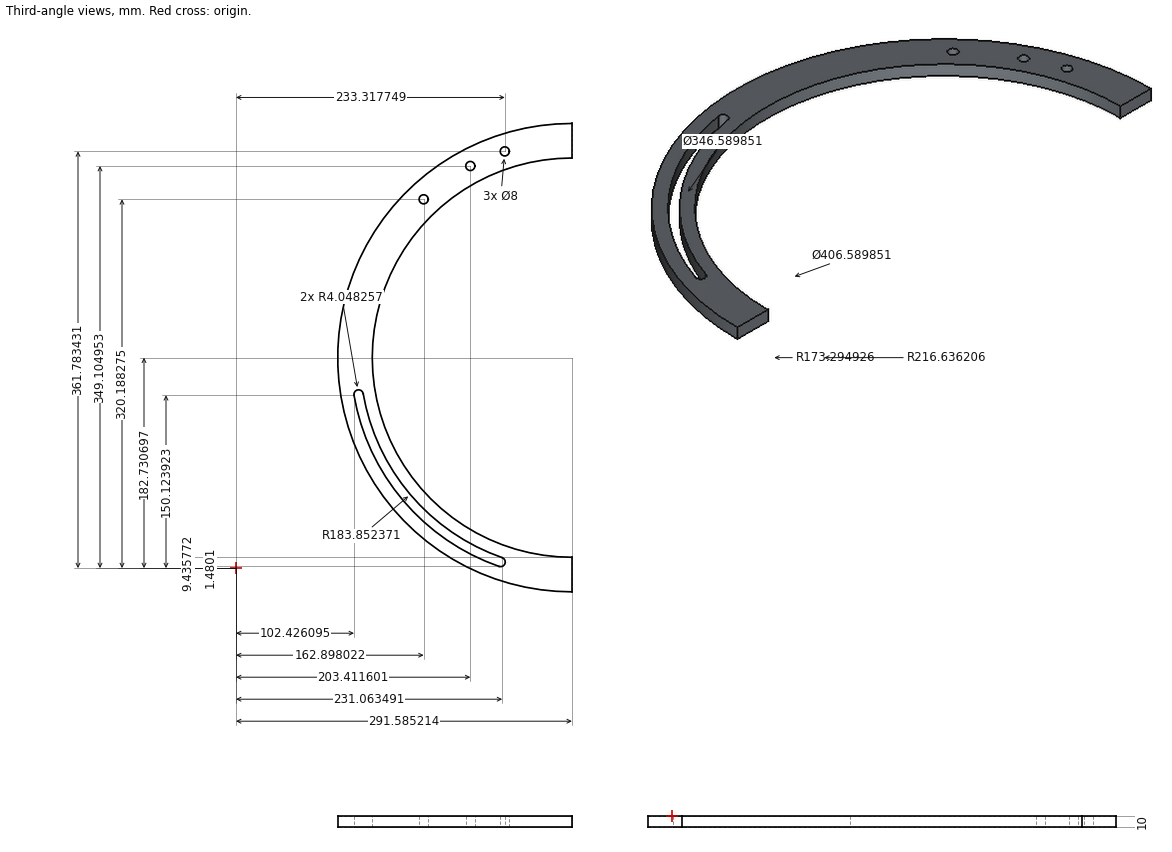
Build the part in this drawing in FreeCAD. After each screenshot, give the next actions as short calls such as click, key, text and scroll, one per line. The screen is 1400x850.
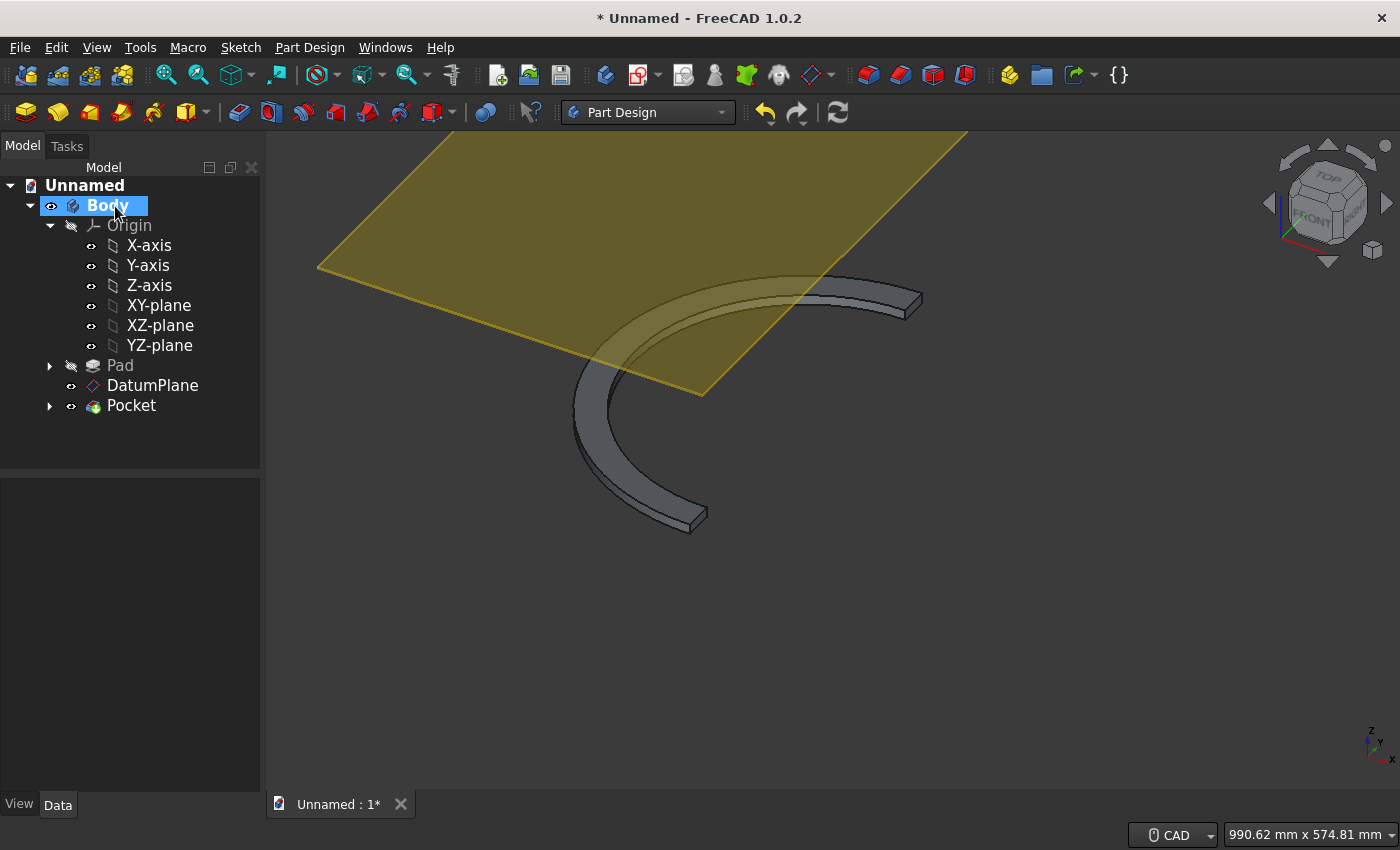
click(116, 386)
key(space)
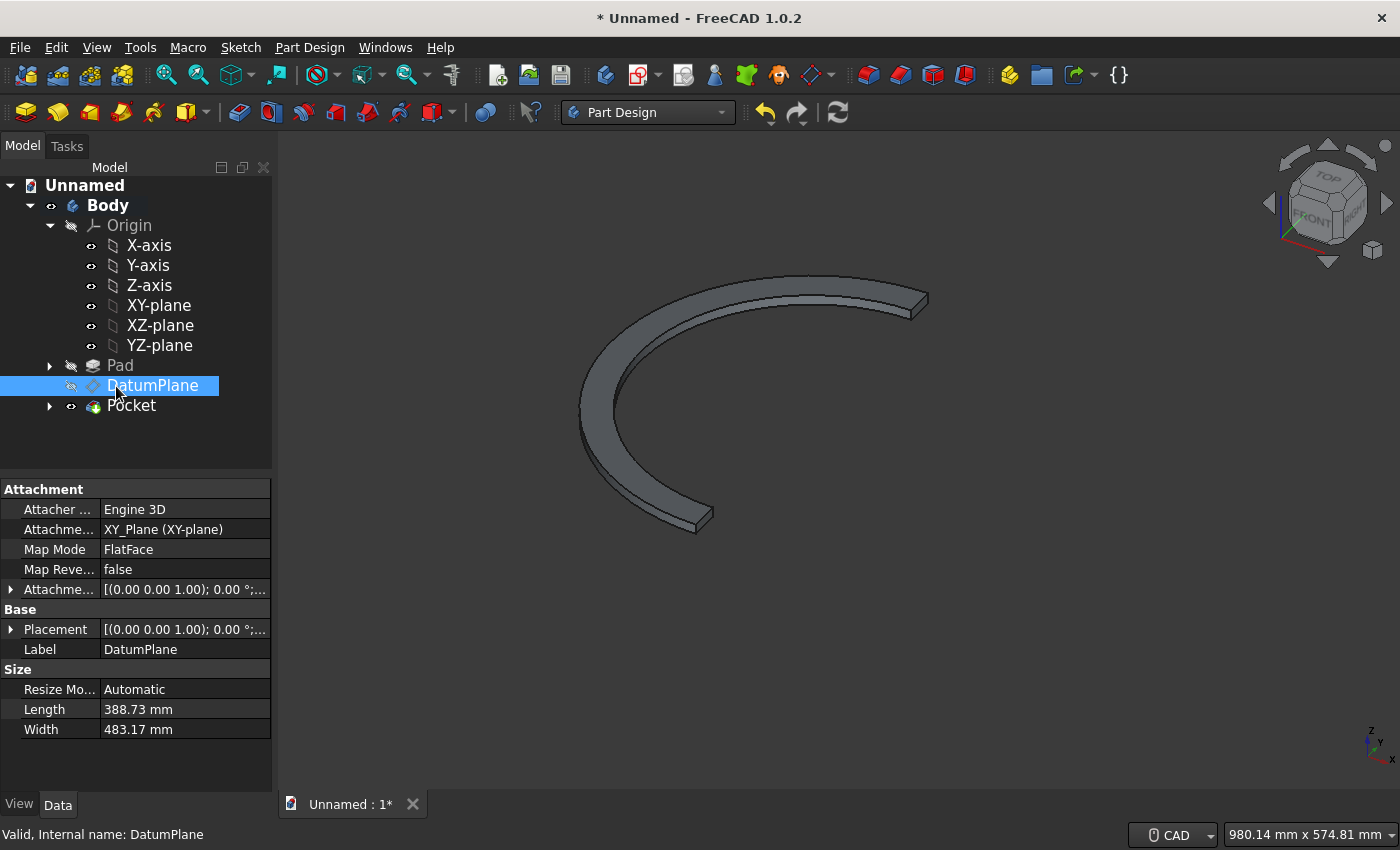
key(5)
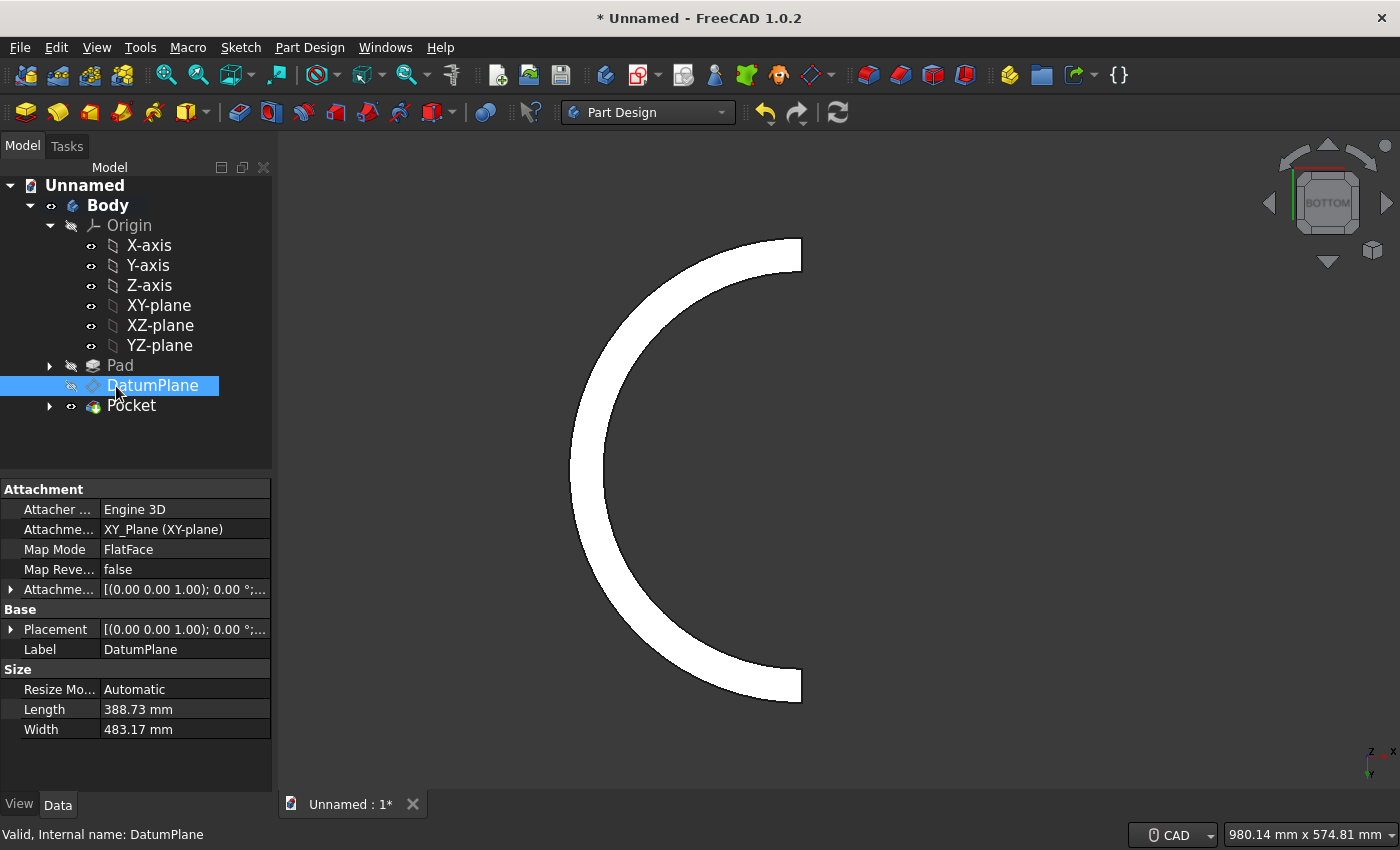
click(719, 669)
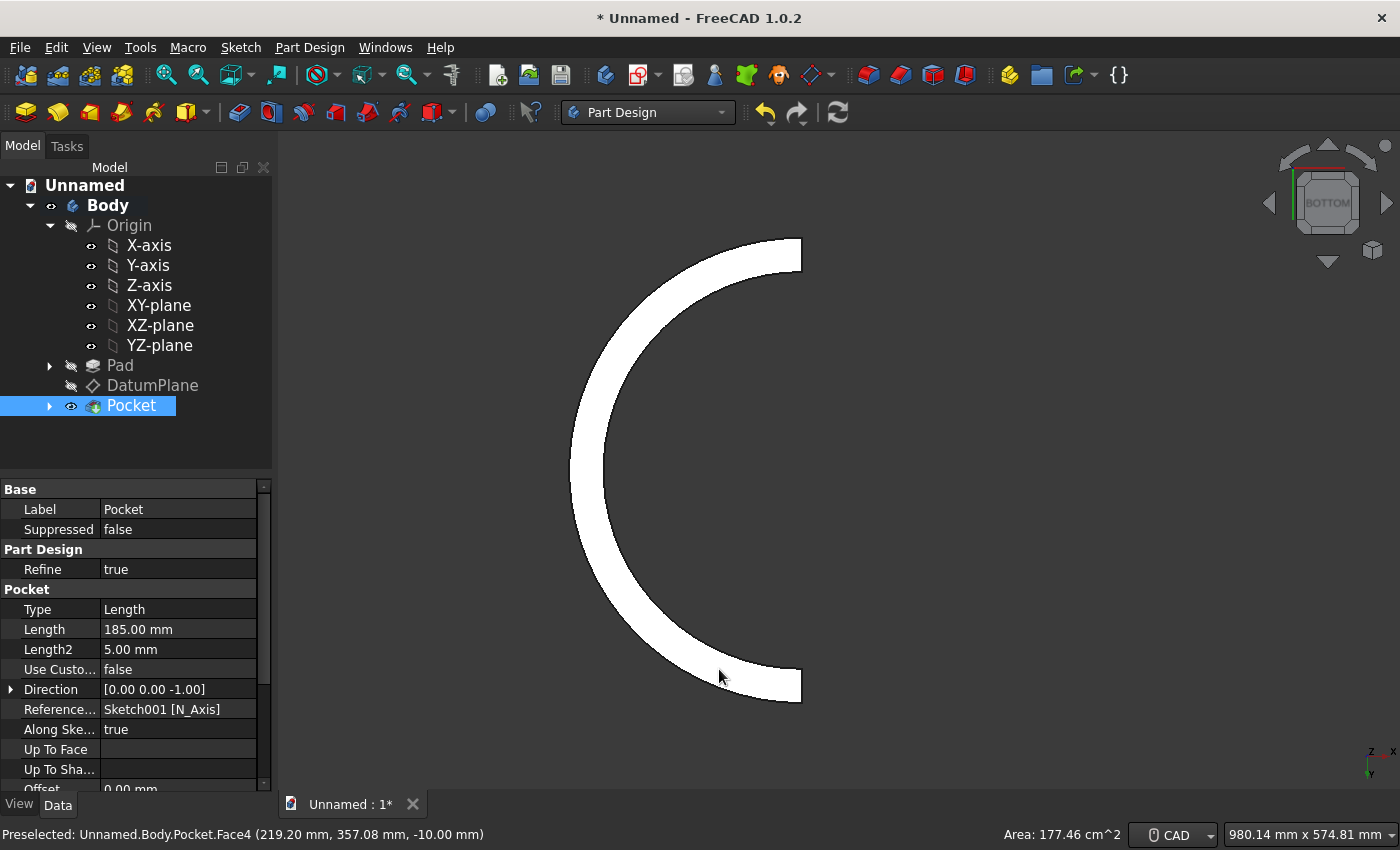
click(638, 76)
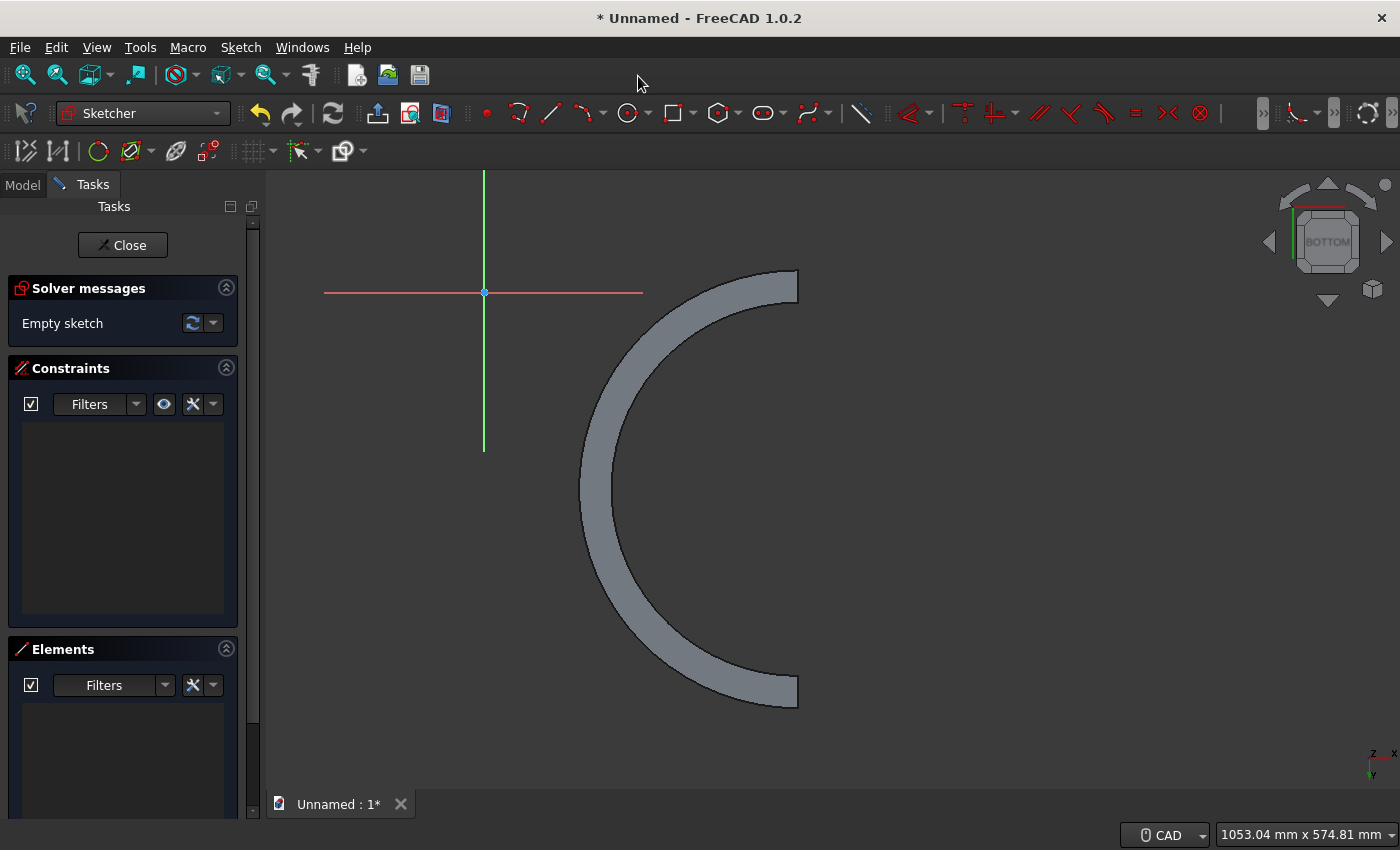
scroll(484, 291, up, 4)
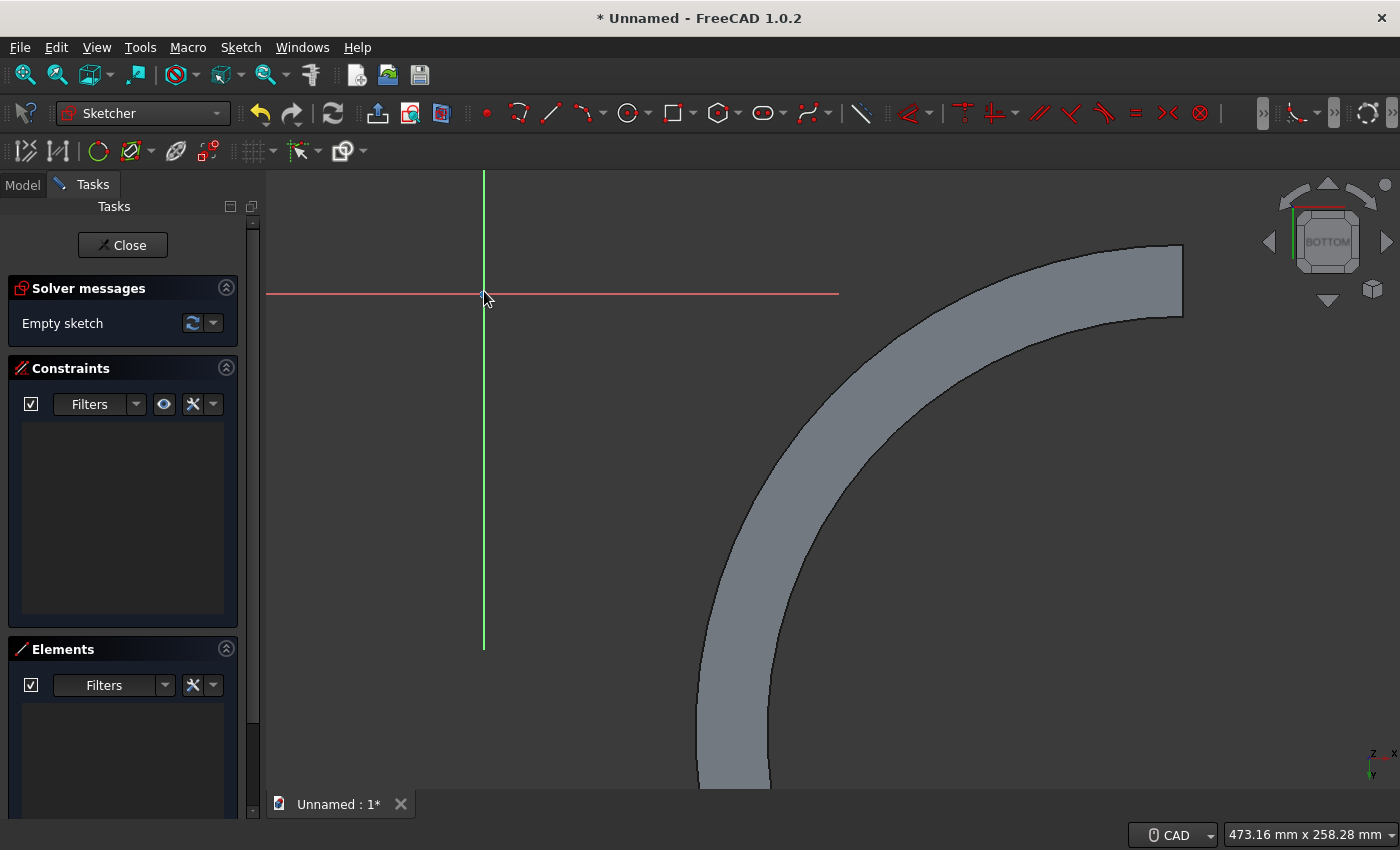
click(584, 114)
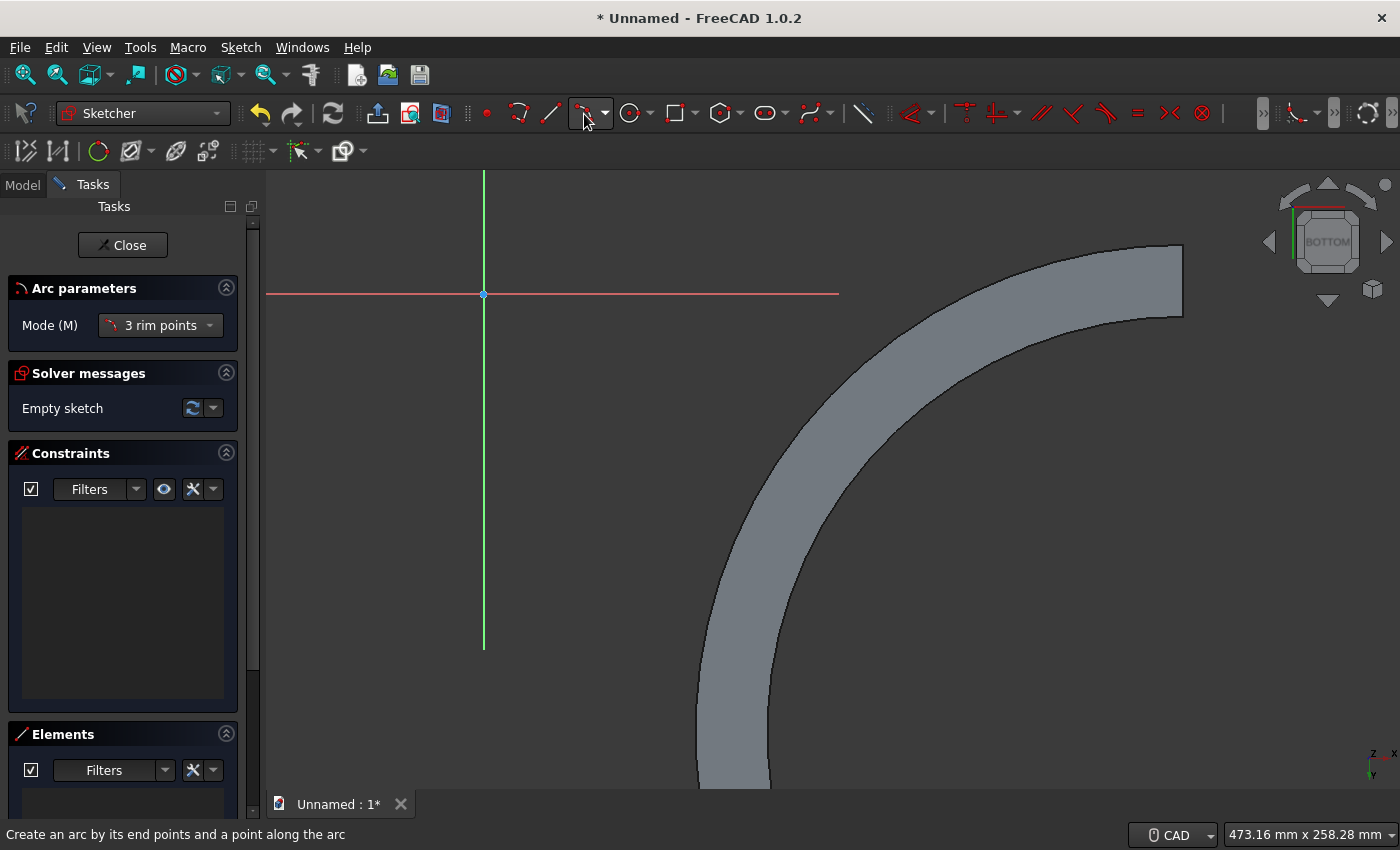
click(729, 654)
click(748, 657)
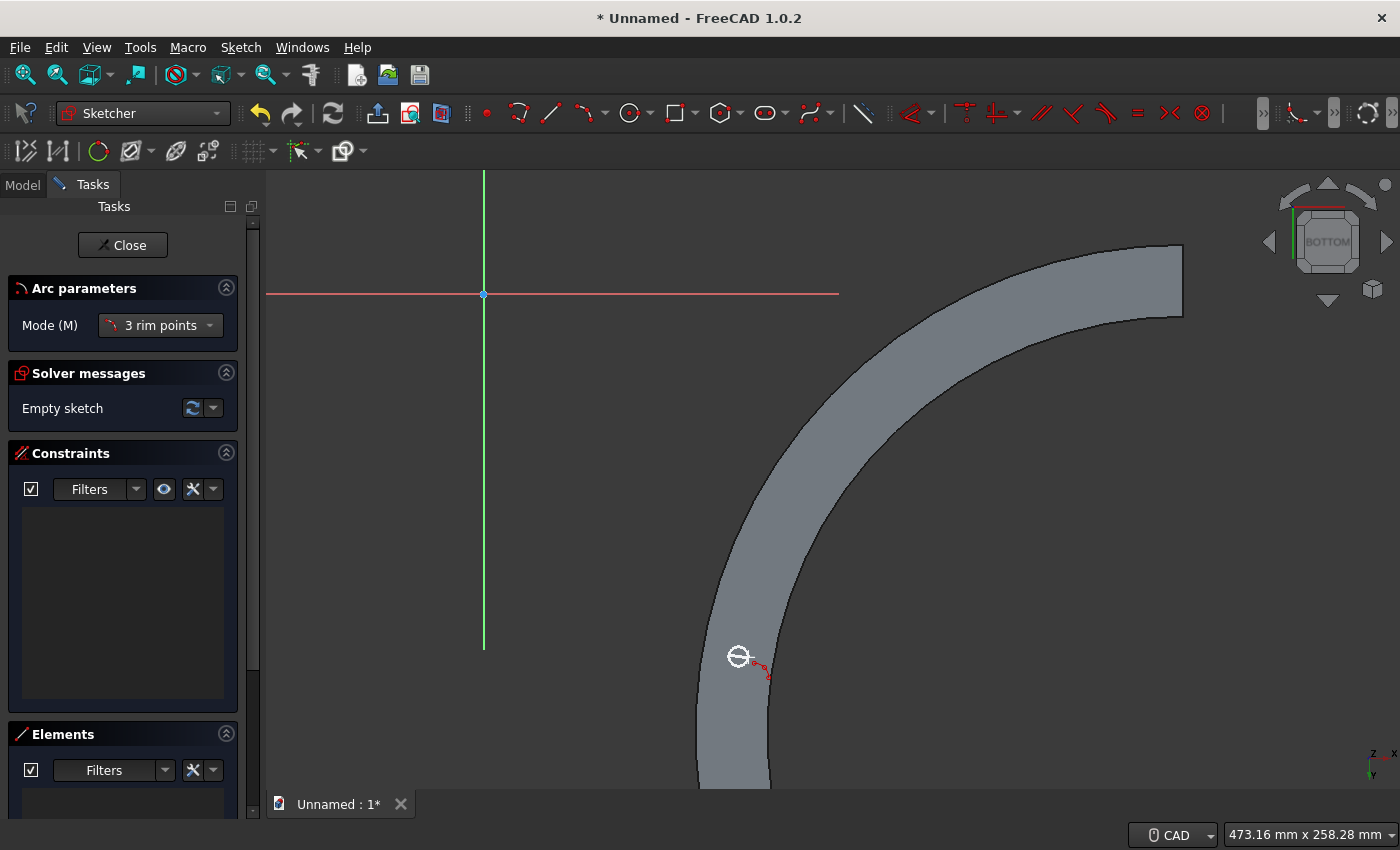
scroll(737, 665, up, 3)